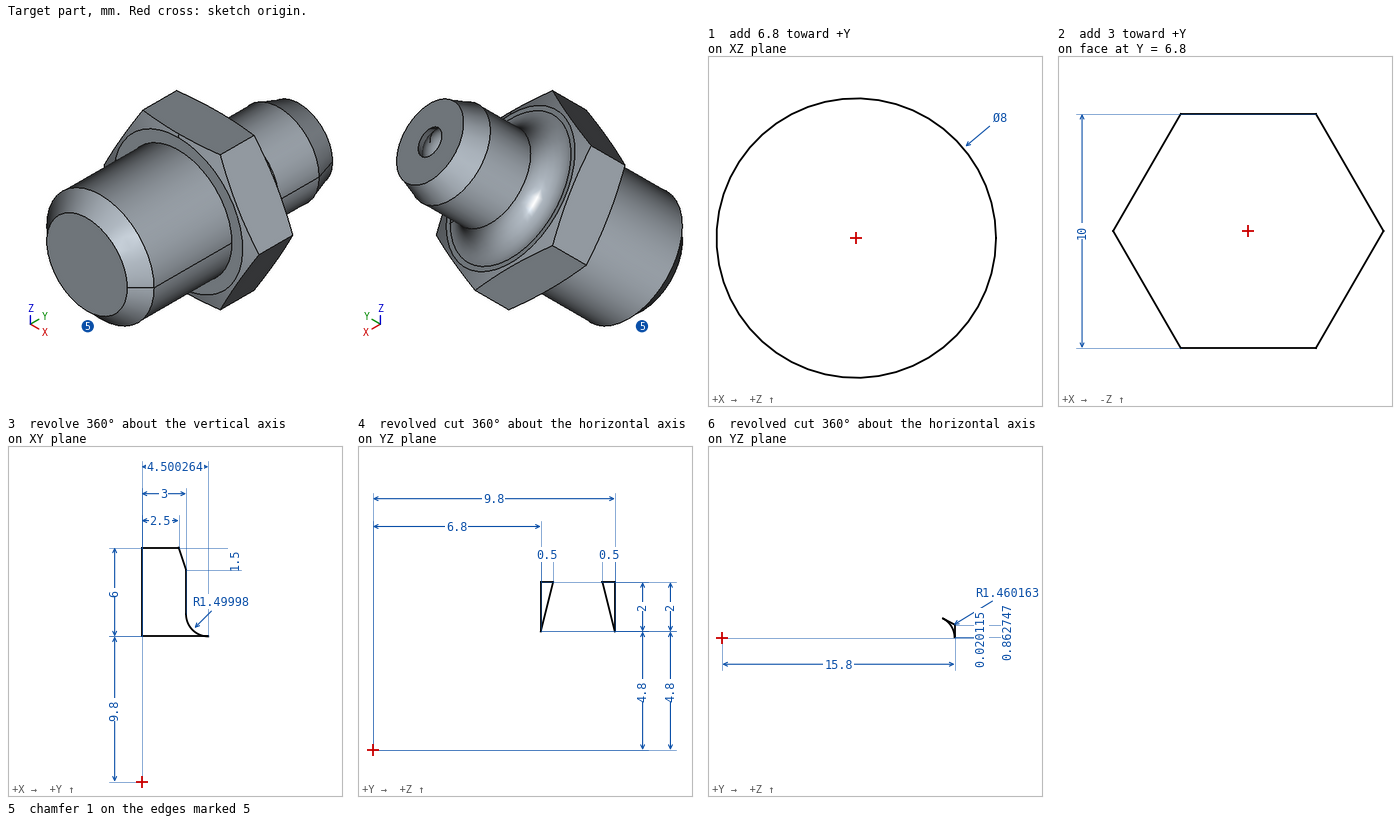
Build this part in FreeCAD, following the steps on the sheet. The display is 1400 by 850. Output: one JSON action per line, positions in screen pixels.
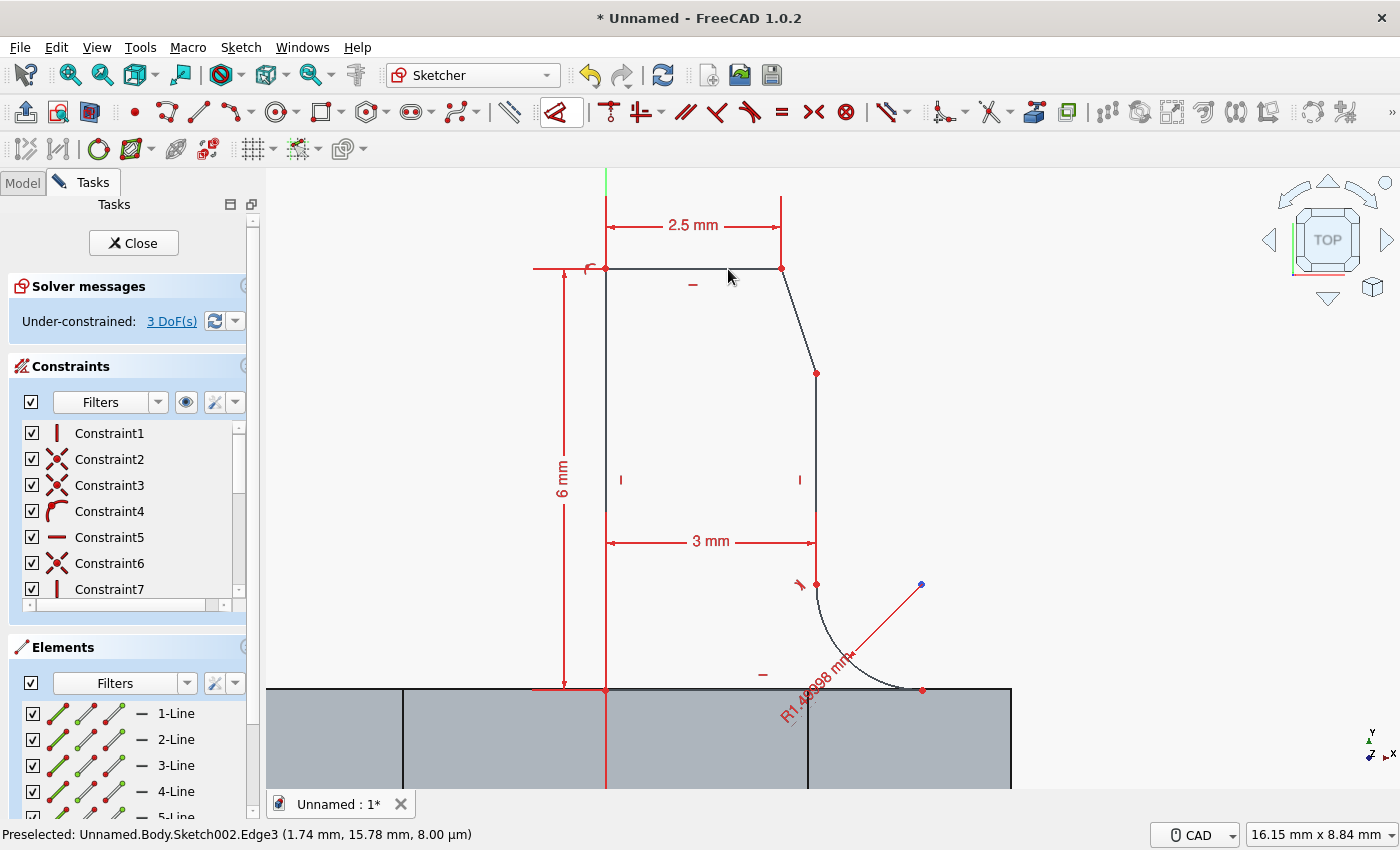
{"action": "left_click", "coordinate": [606, 690]}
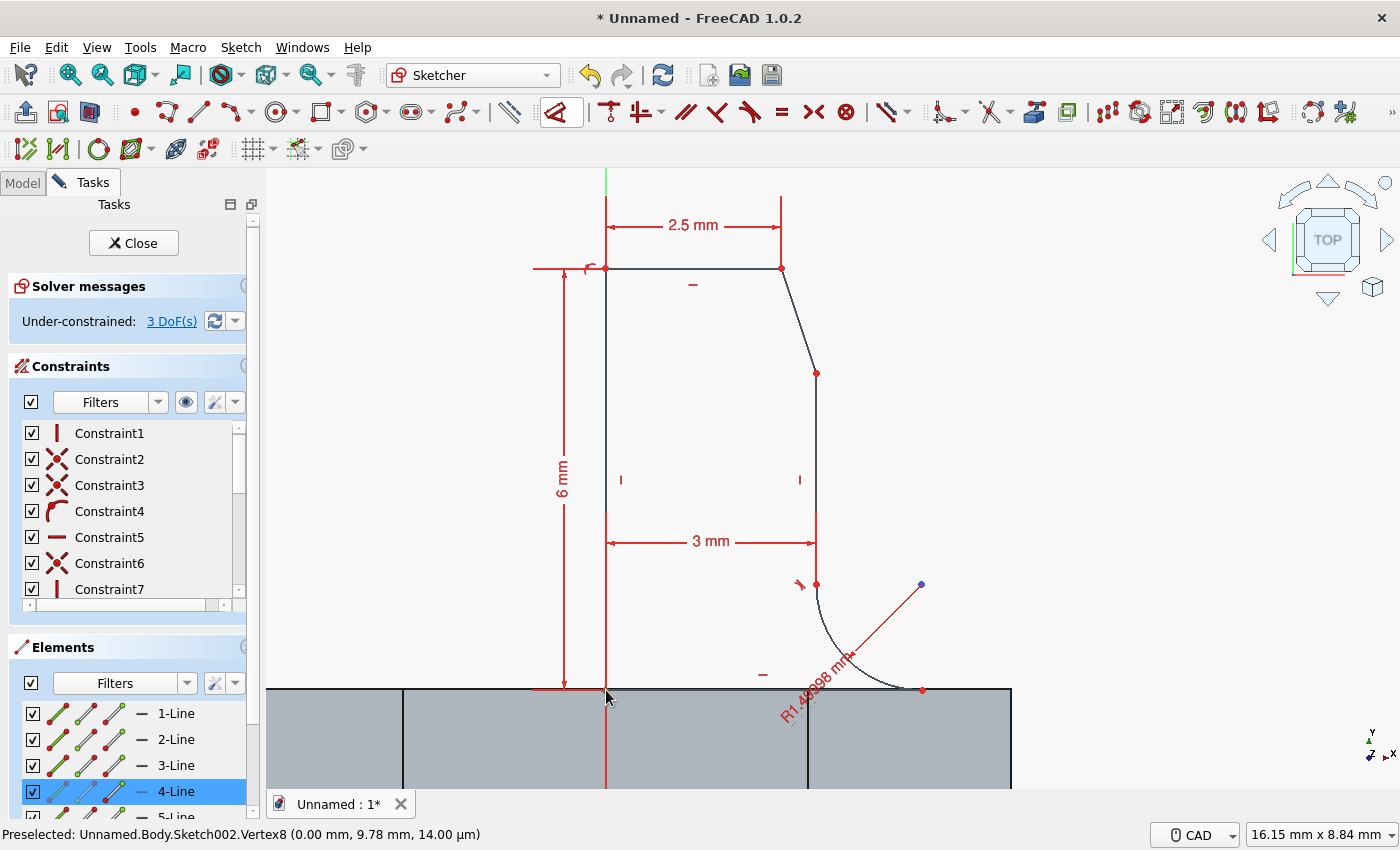
{"action": "key", "text": "i"}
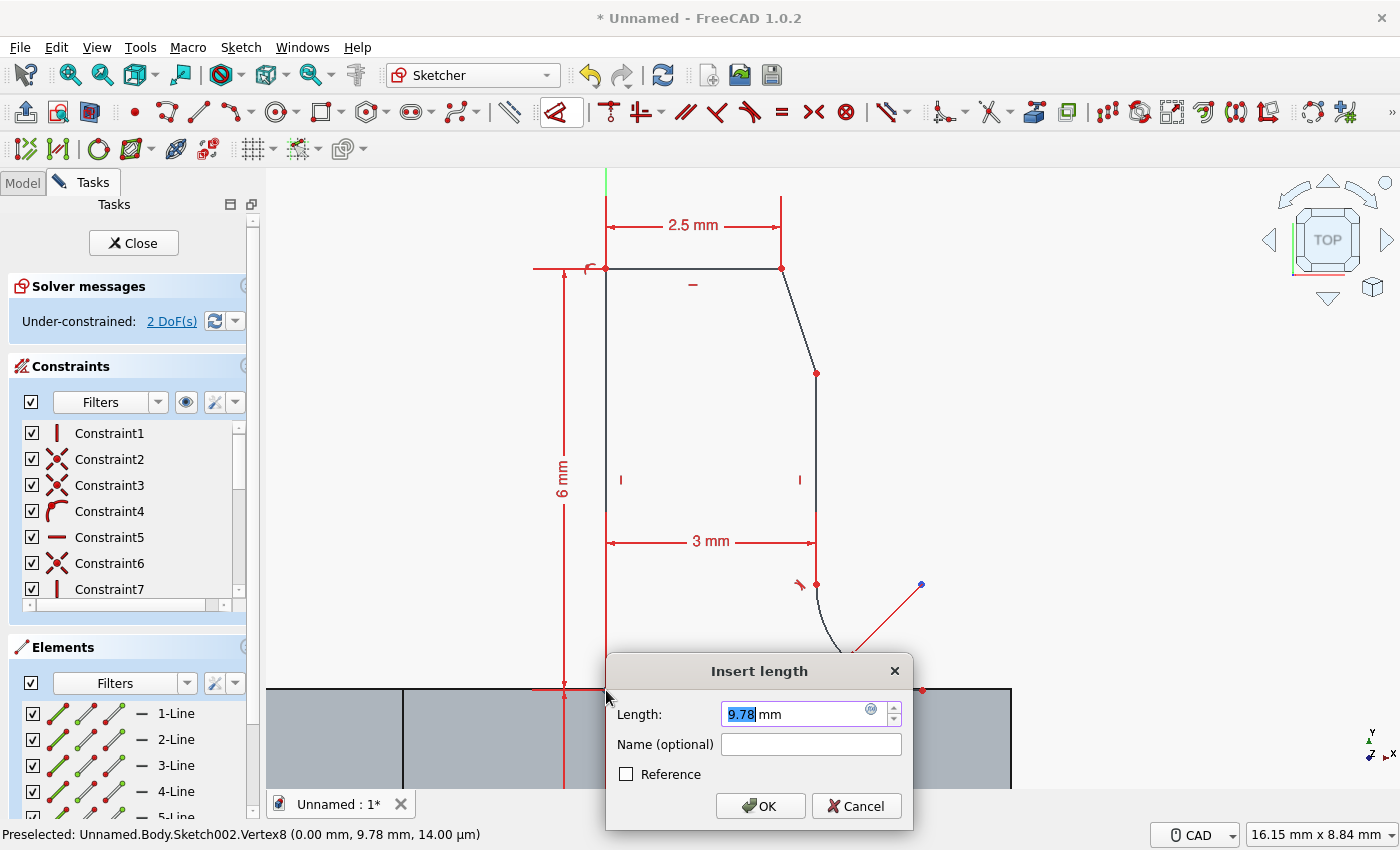
{"action": "type", "text": "9.8"}
{"action": "key", "text": "Return"}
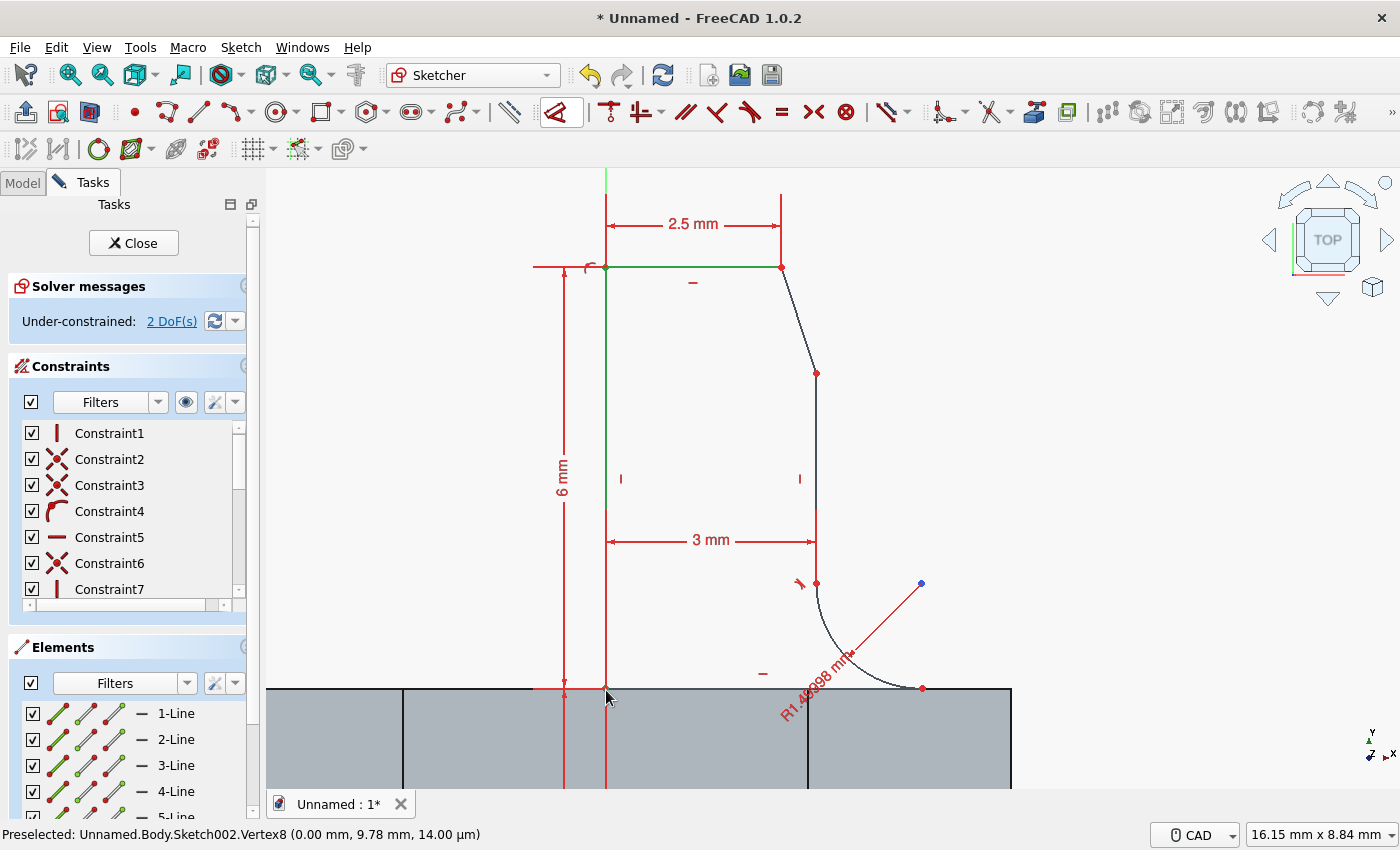
{"action": "left_click", "coordinate": [806, 342]}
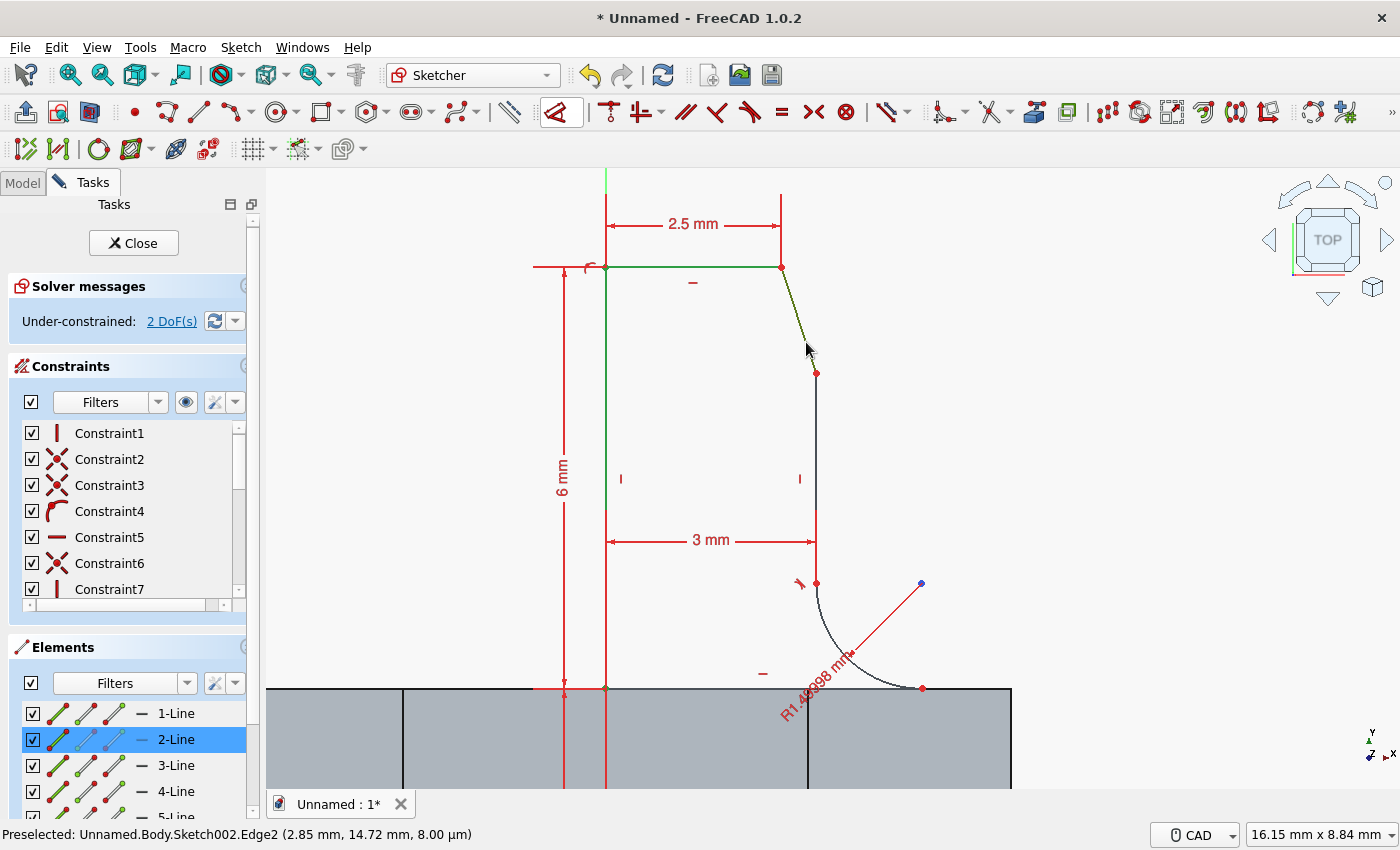
{"action": "key", "text": "i"}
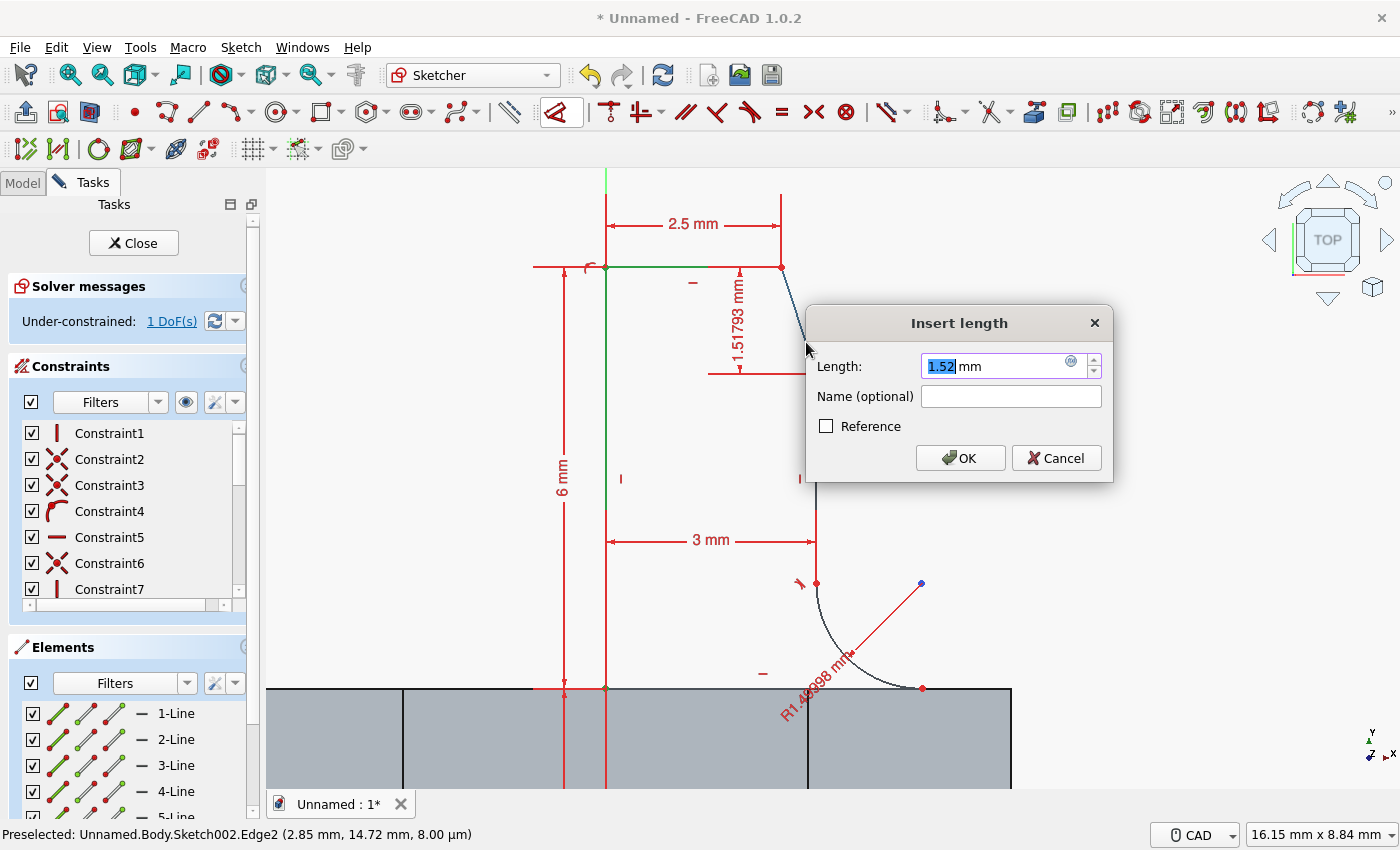
{"action": "type", "text": "1.5"}
{"action": "key", "text": "Return"}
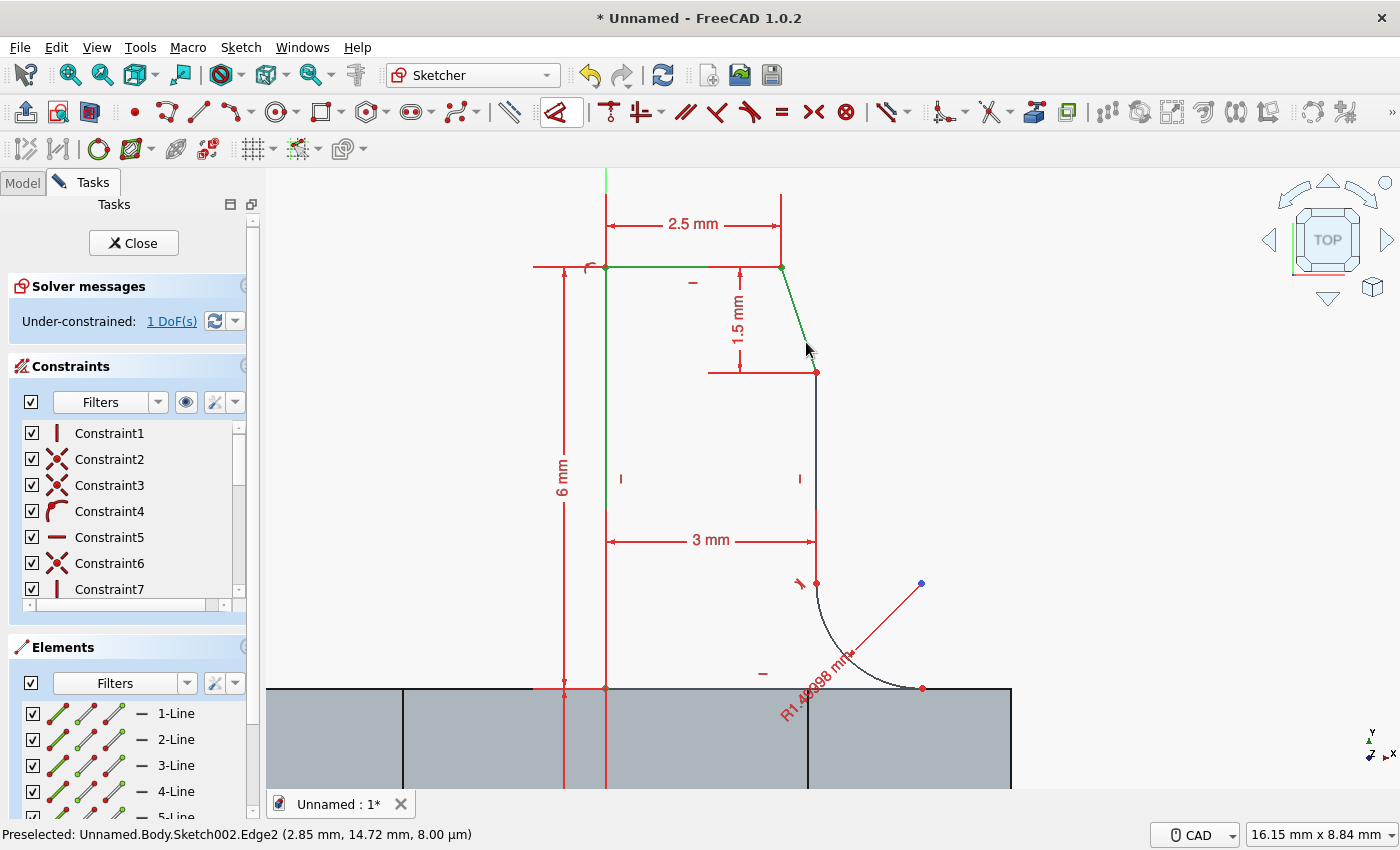
{"action": "left_click", "coordinate": [701, 689]}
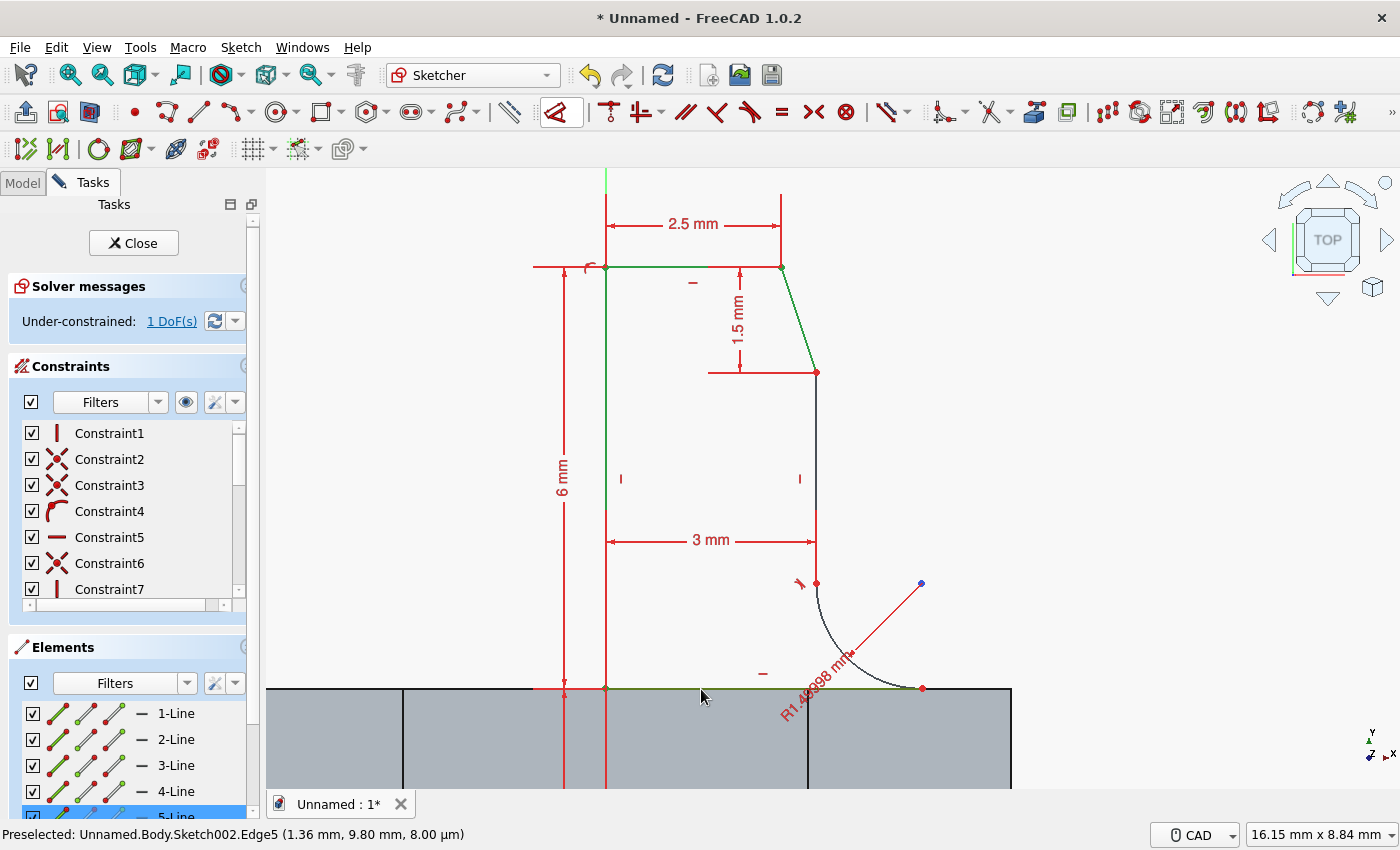
{"action": "key", "text": "l"}